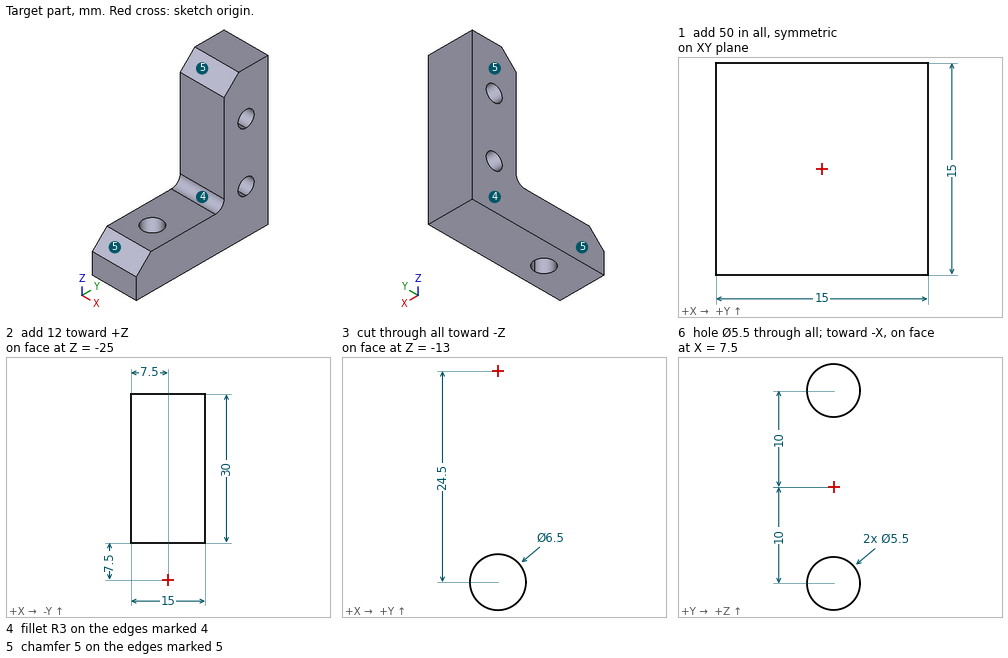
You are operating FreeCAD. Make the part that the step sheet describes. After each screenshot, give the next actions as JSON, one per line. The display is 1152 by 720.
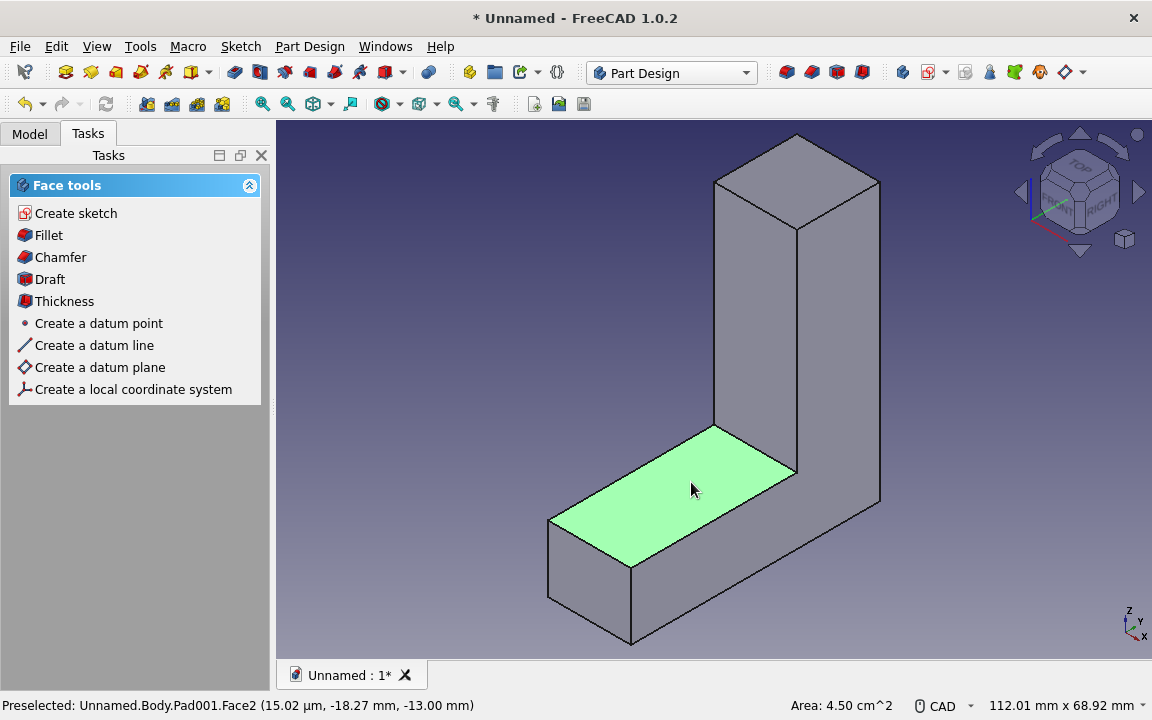
{"action": "left_click", "coordinate": [928, 72]}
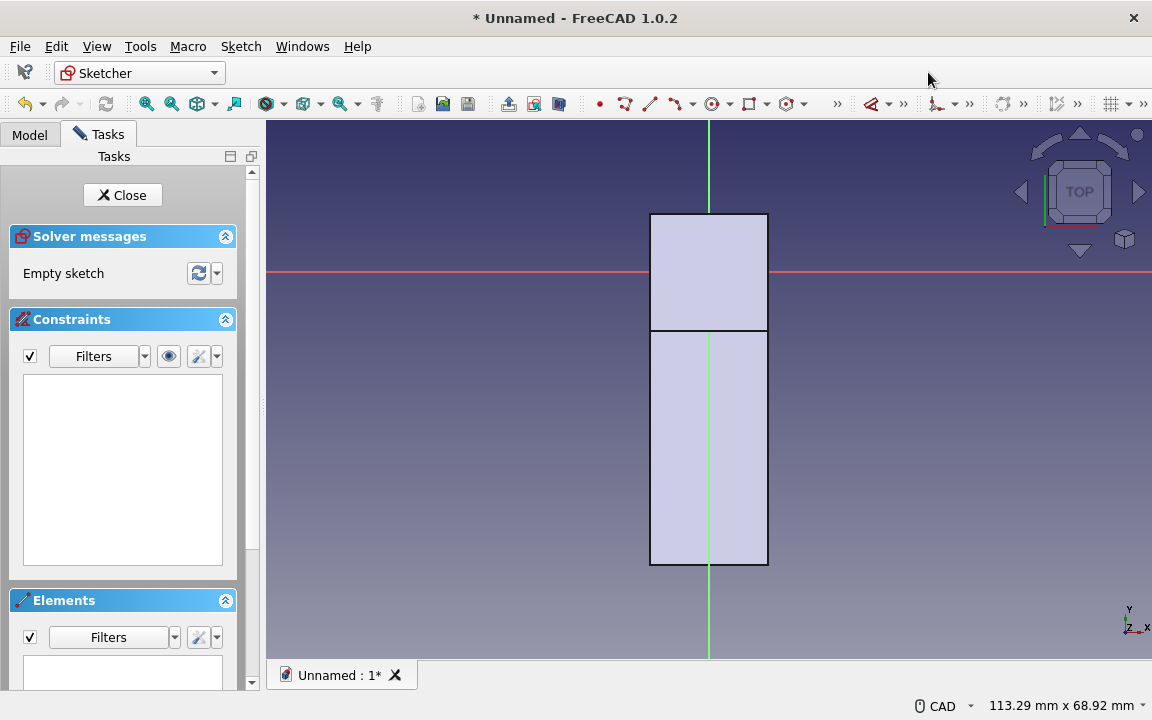
{"action": "key", "text": "q s"}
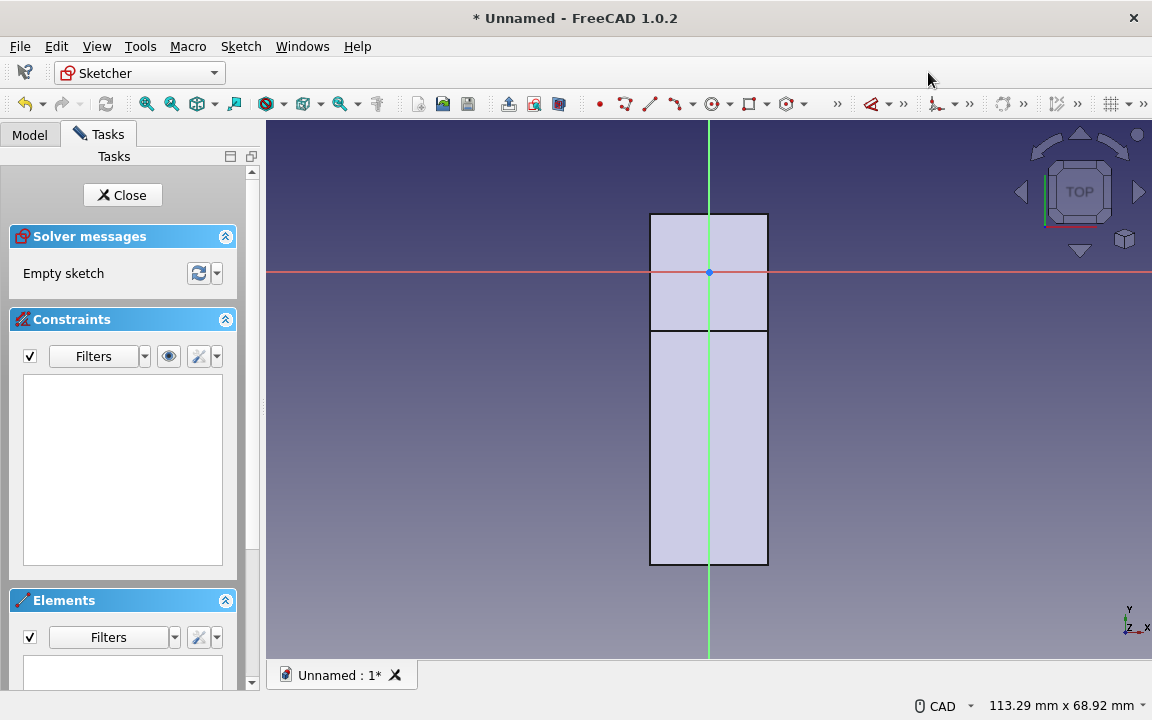
{"action": "scroll", "coordinate": [720, 475], "scroll_direction": "up", "scroll_amount": 10}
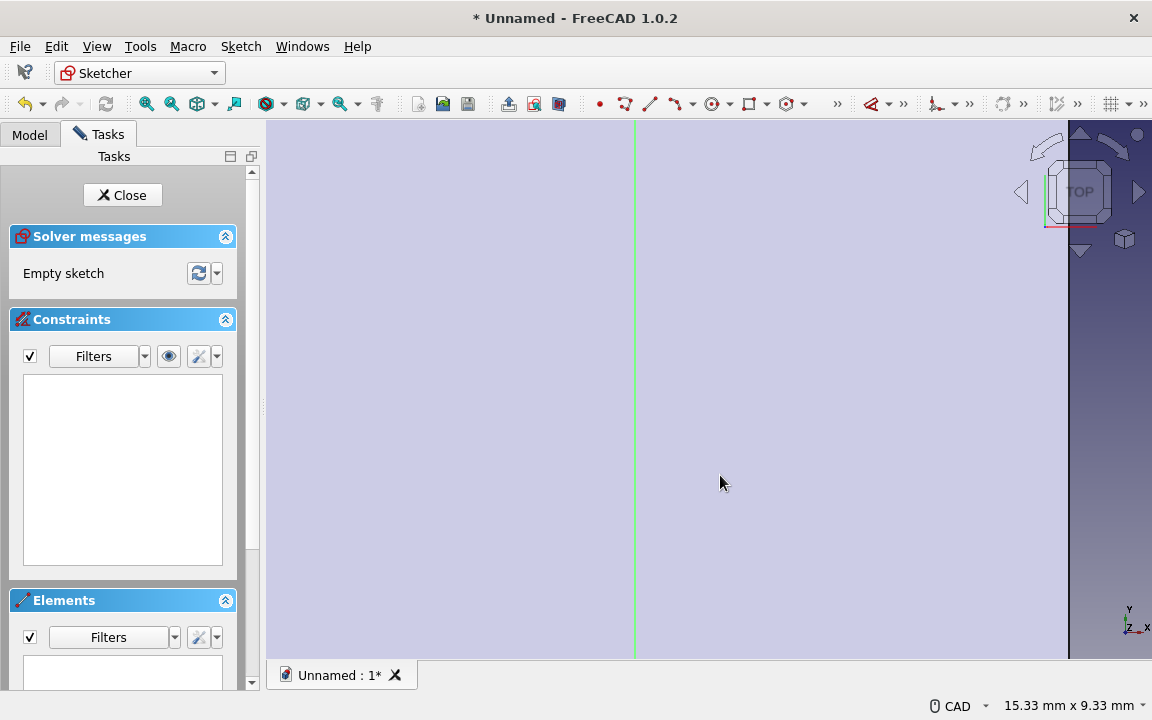
{"action": "key", "text": "g c"}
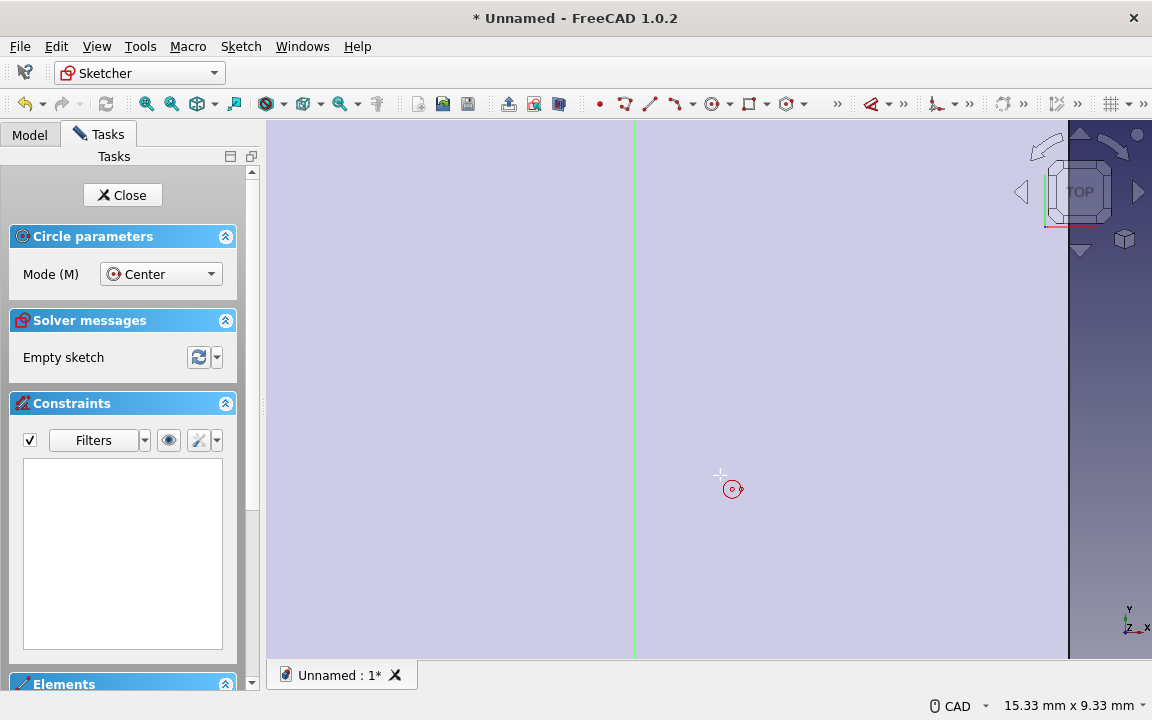
{"action": "left_click", "coordinate": [635, 388]}
{"action": "mouse_move", "coordinate": [768, 255]}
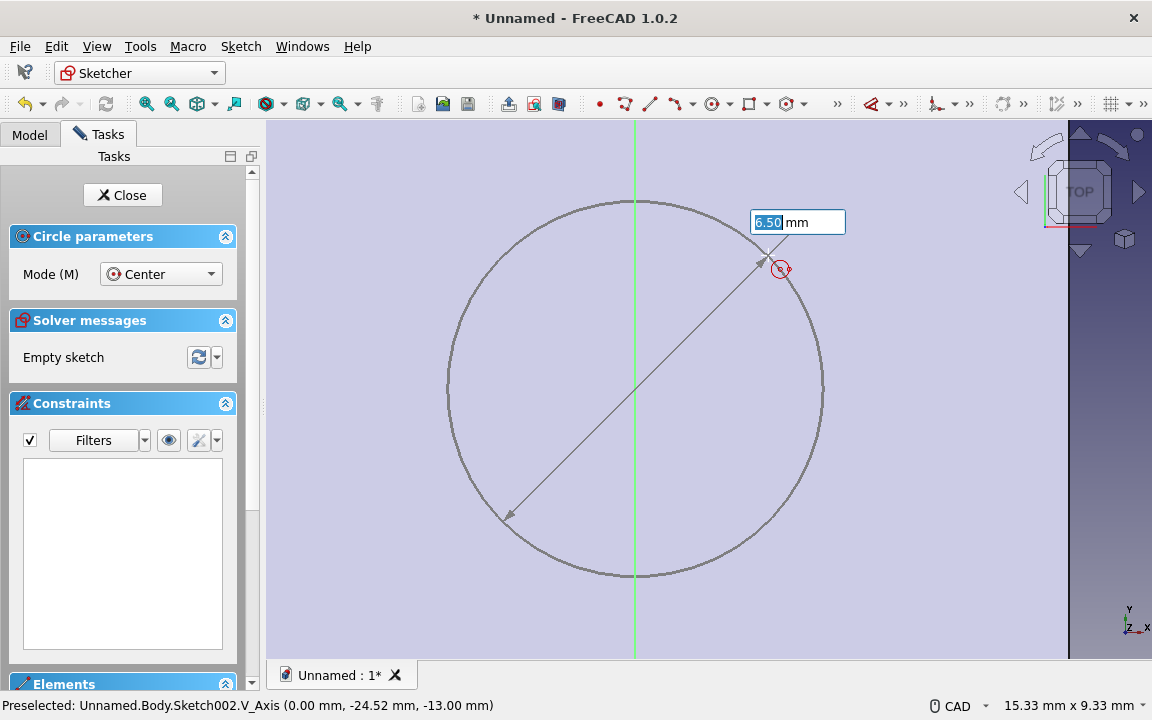
{"action": "type", "text": "6.5"}
{"action": "key", "text": "Return"}
{"action": "key", "text": "Escape"}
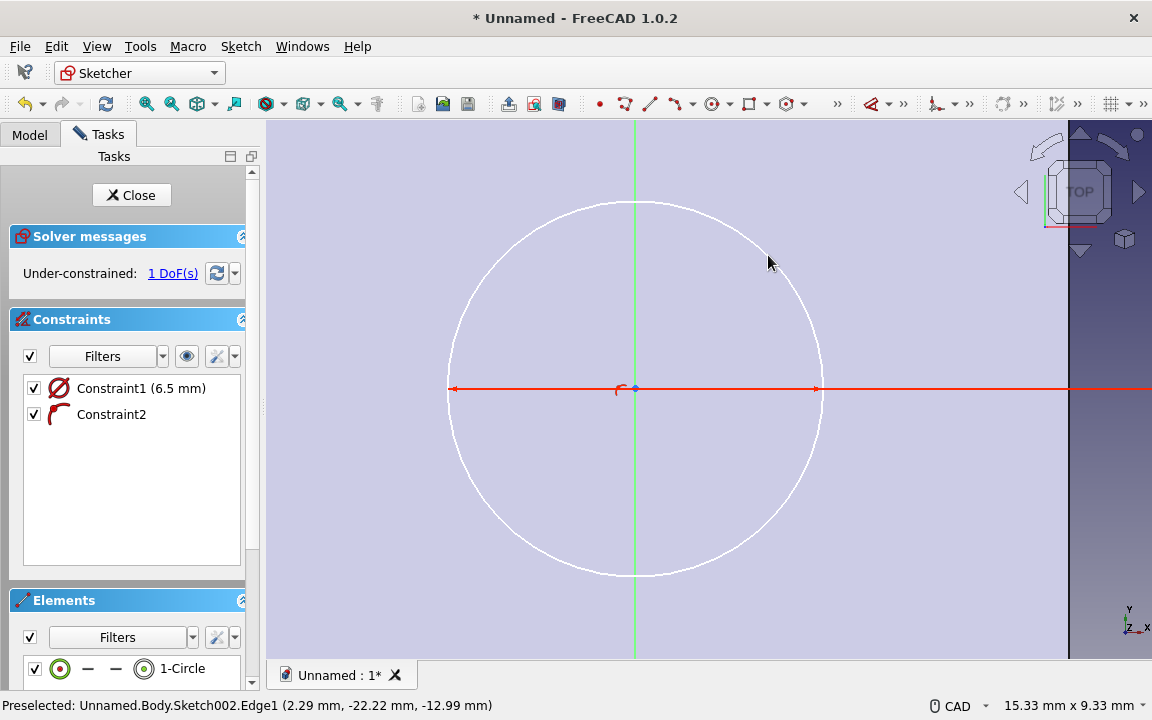
{"action": "left_click", "coordinate": [635, 389]}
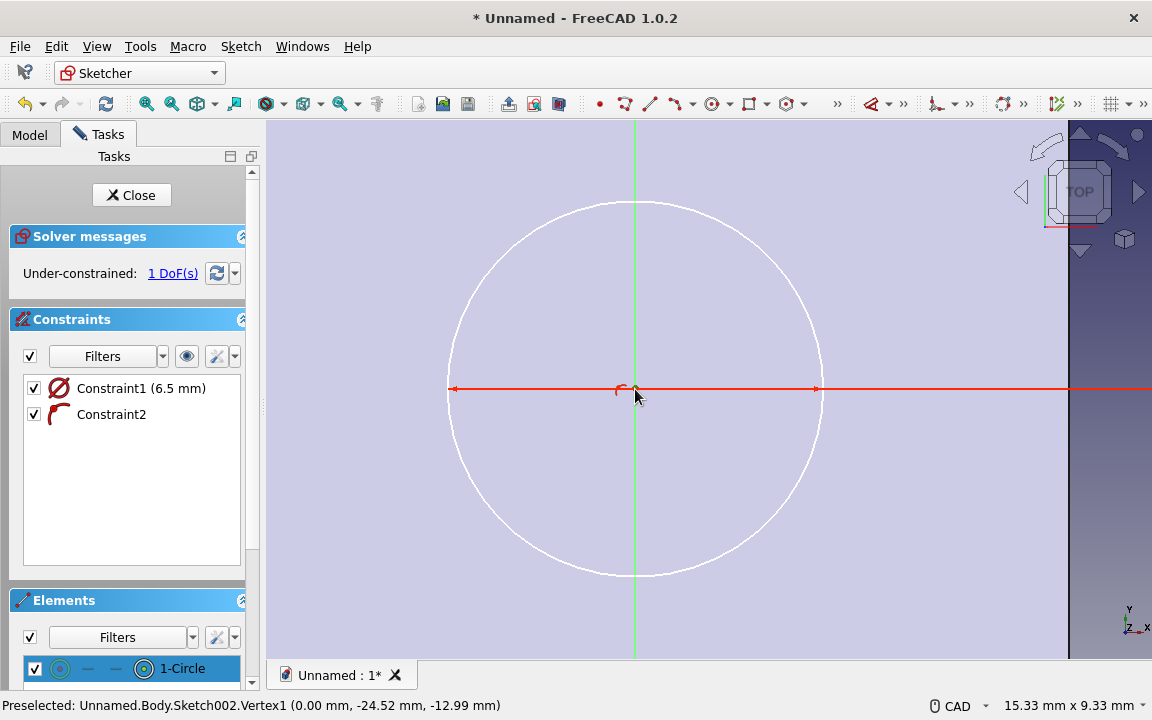
{"action": "key", "text": "i"}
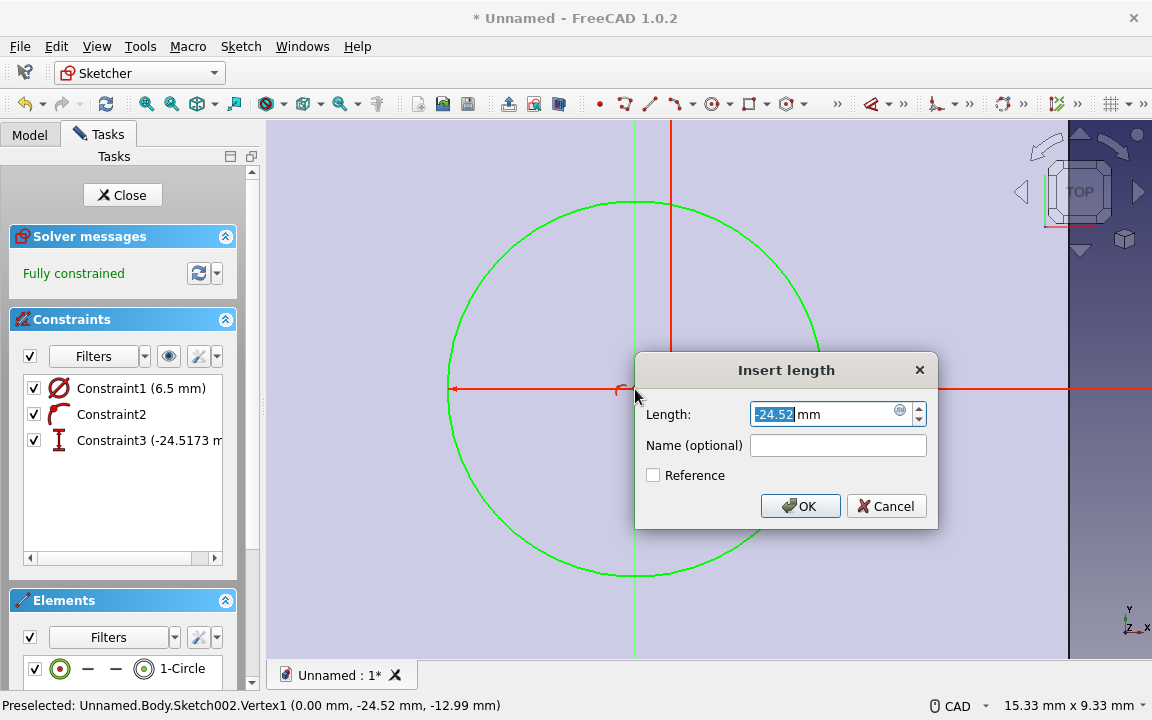
{"action": "type", "text": "-24.5"}
{"action": "key", "text": "Return"}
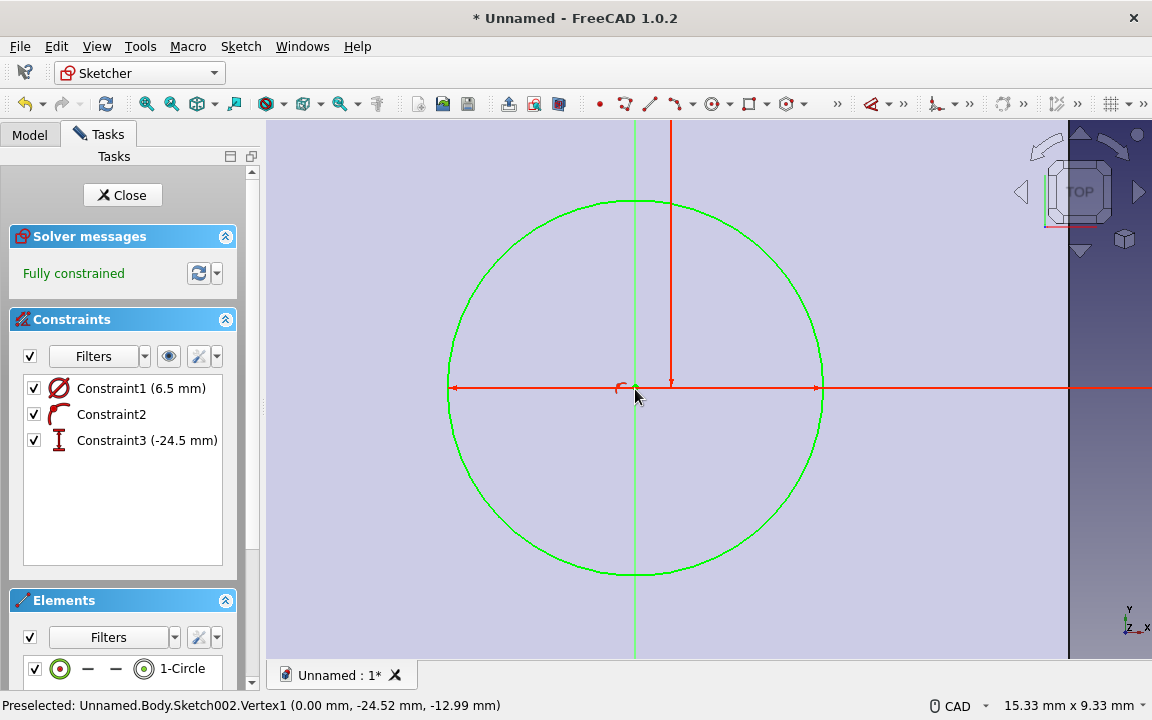
{"action": "left_click", "coordinate": [123, 195]}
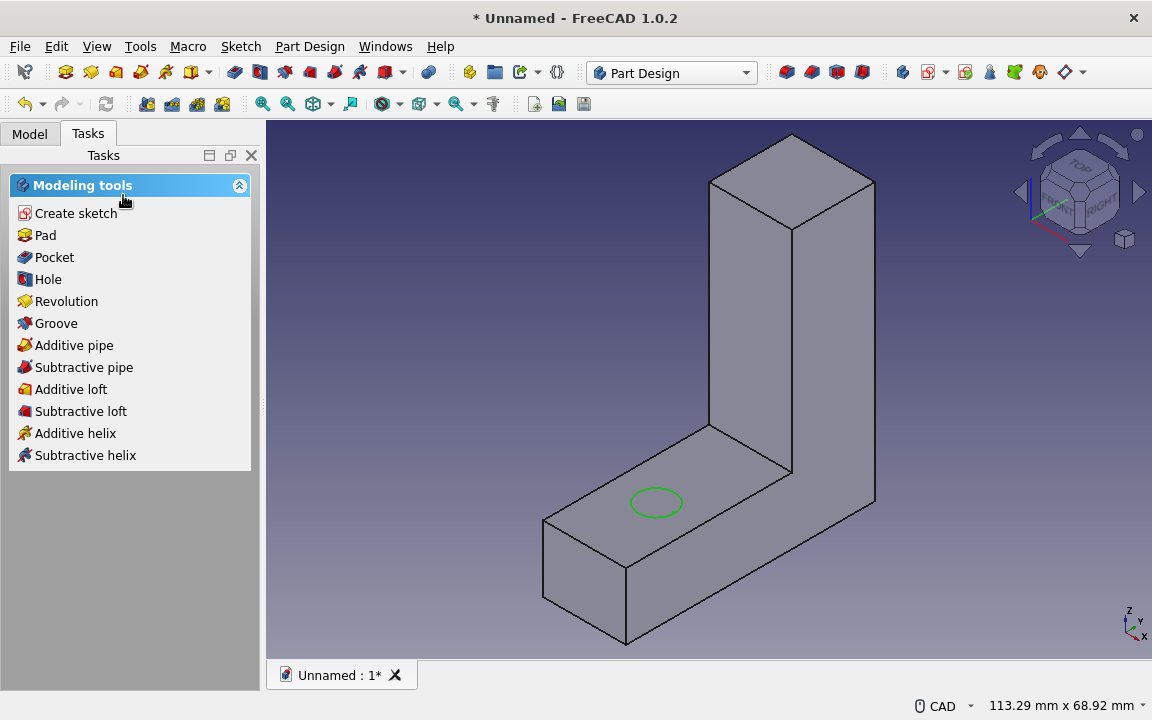
{"action": "left_click", "coordinate": [235, 72]}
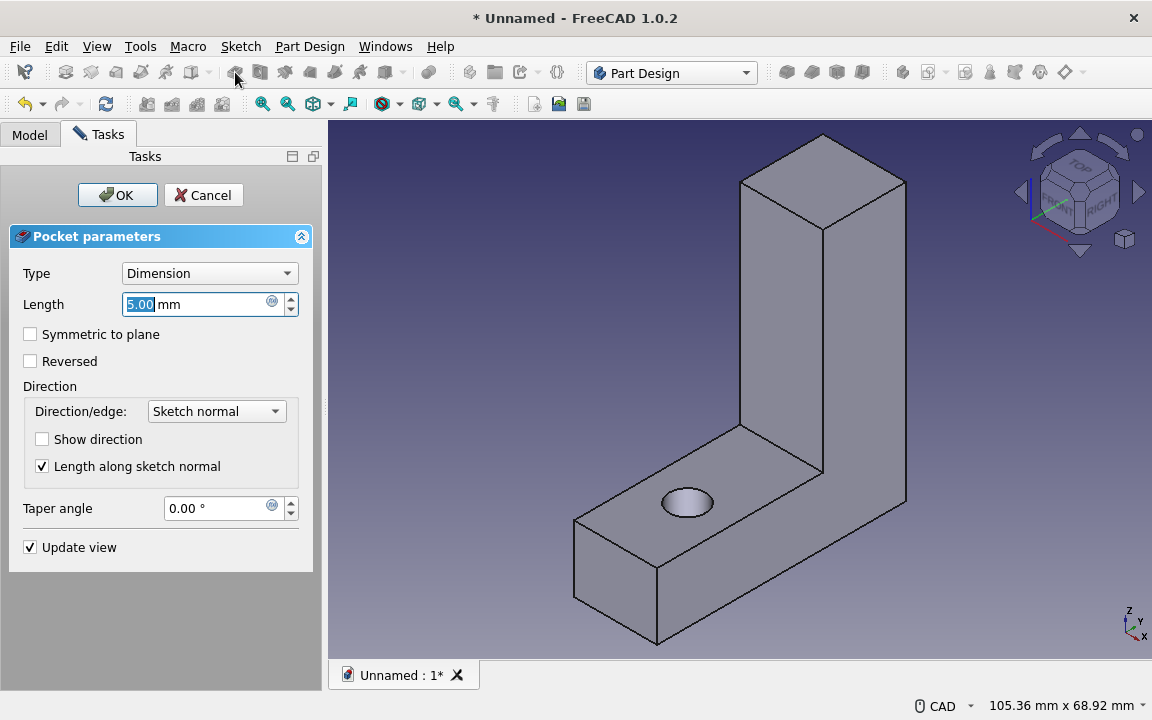
{"action": "left_click", "coordinate": [210, 274]}